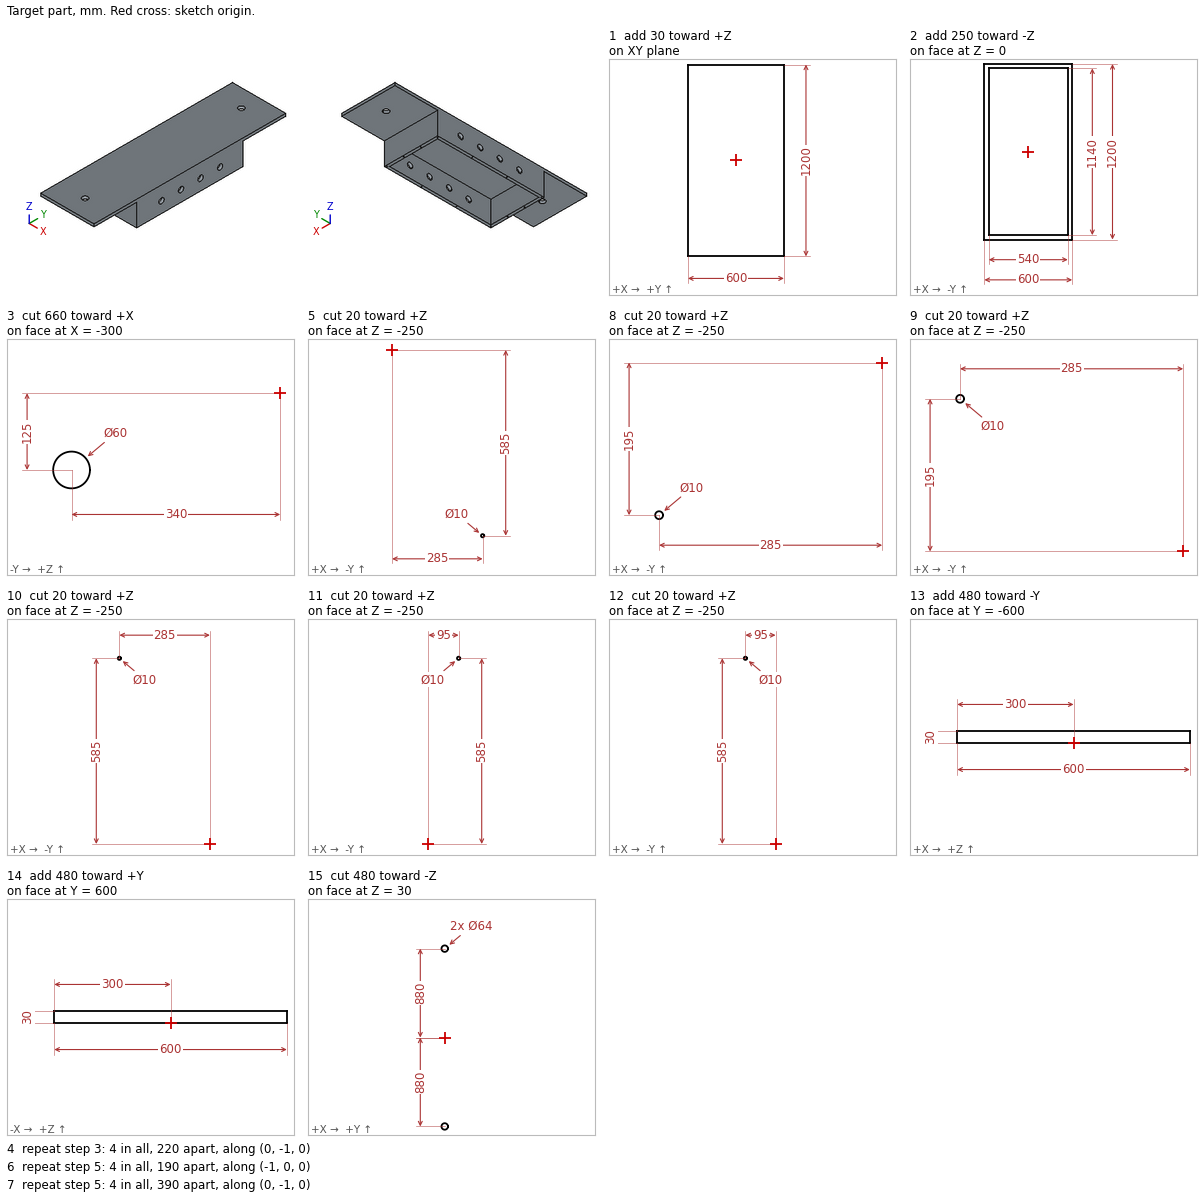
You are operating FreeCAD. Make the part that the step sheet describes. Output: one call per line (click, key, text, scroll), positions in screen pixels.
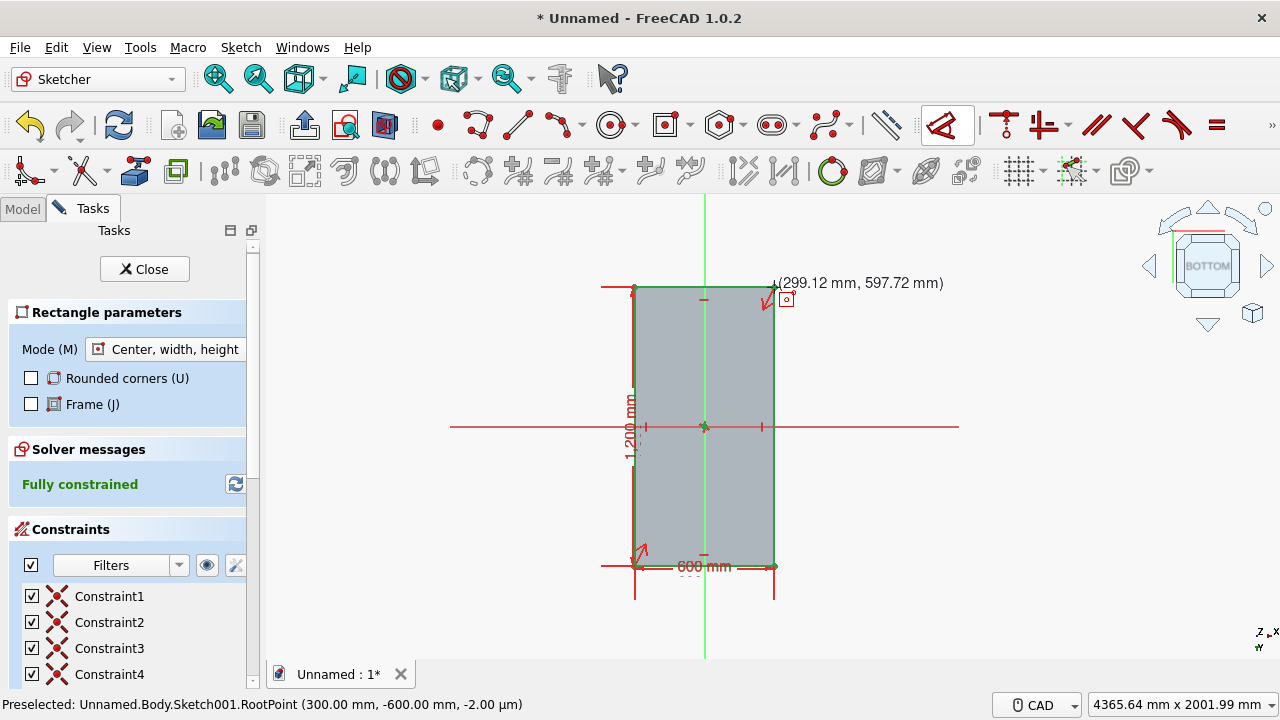
click(705, 427)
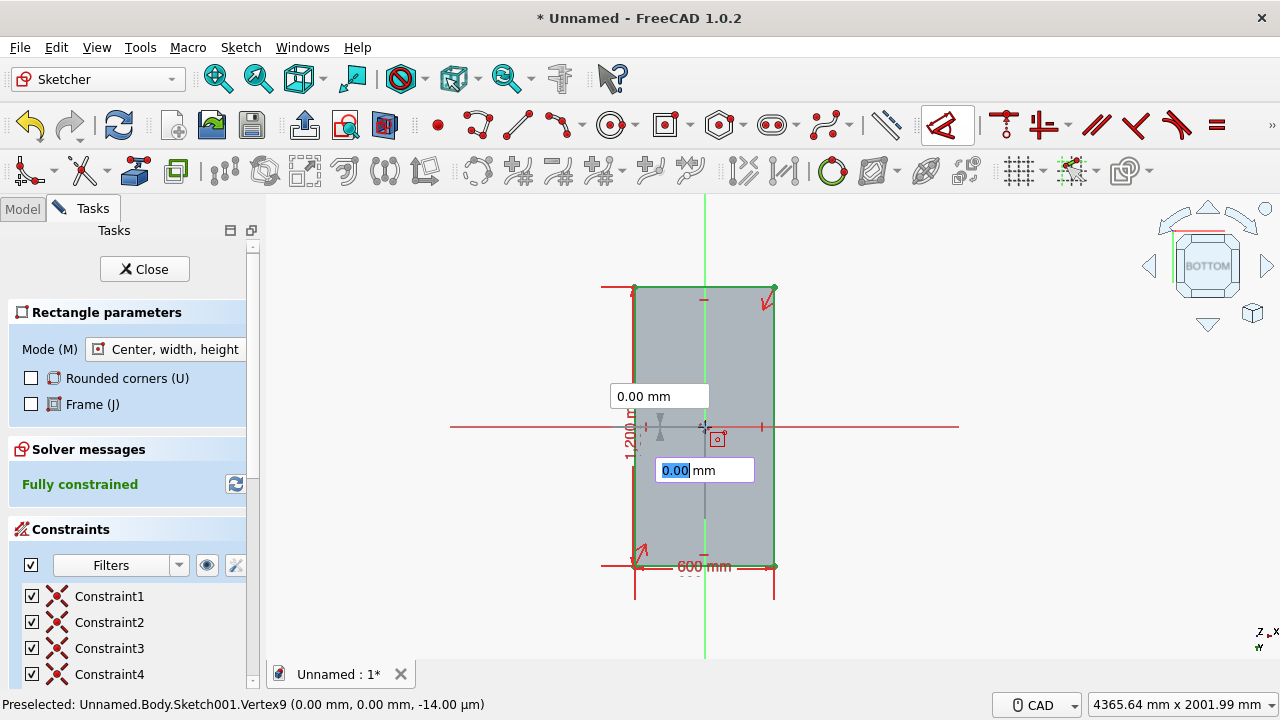
scroll(767, 294, up, 5)
move(767, 295)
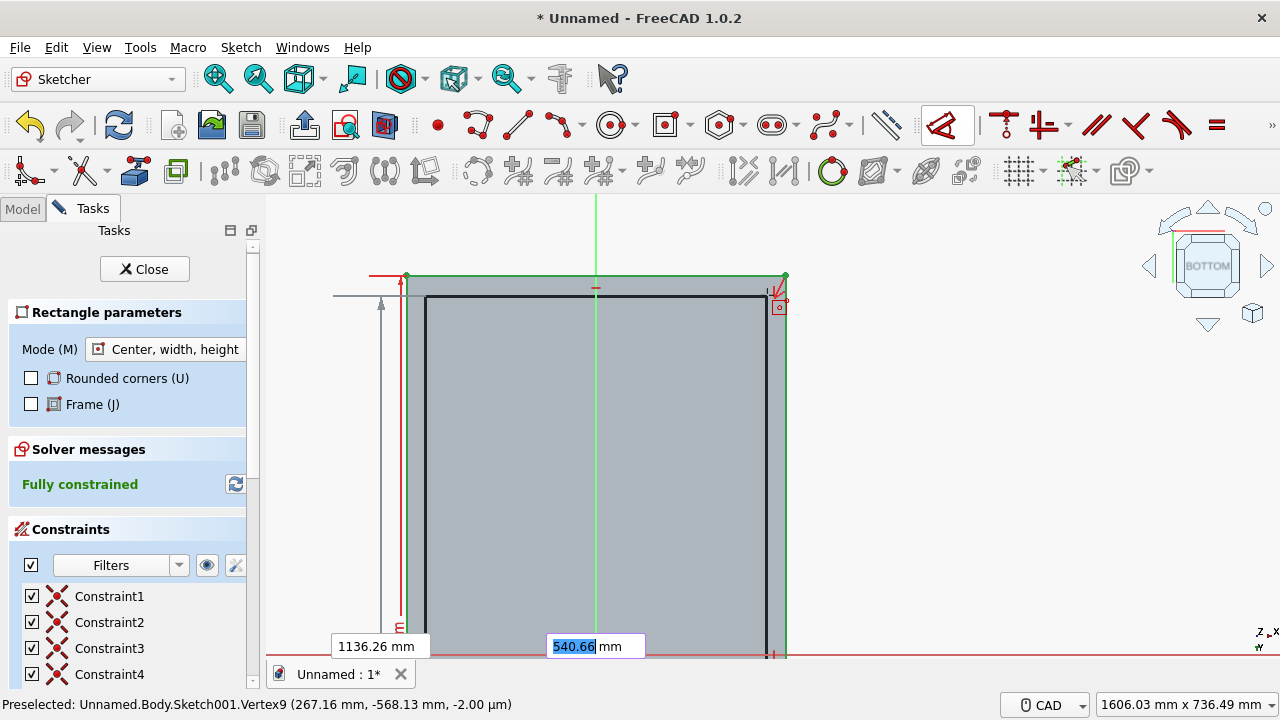
text(540)
key(Tab)
text(1140)
key(Return)
key(Escape)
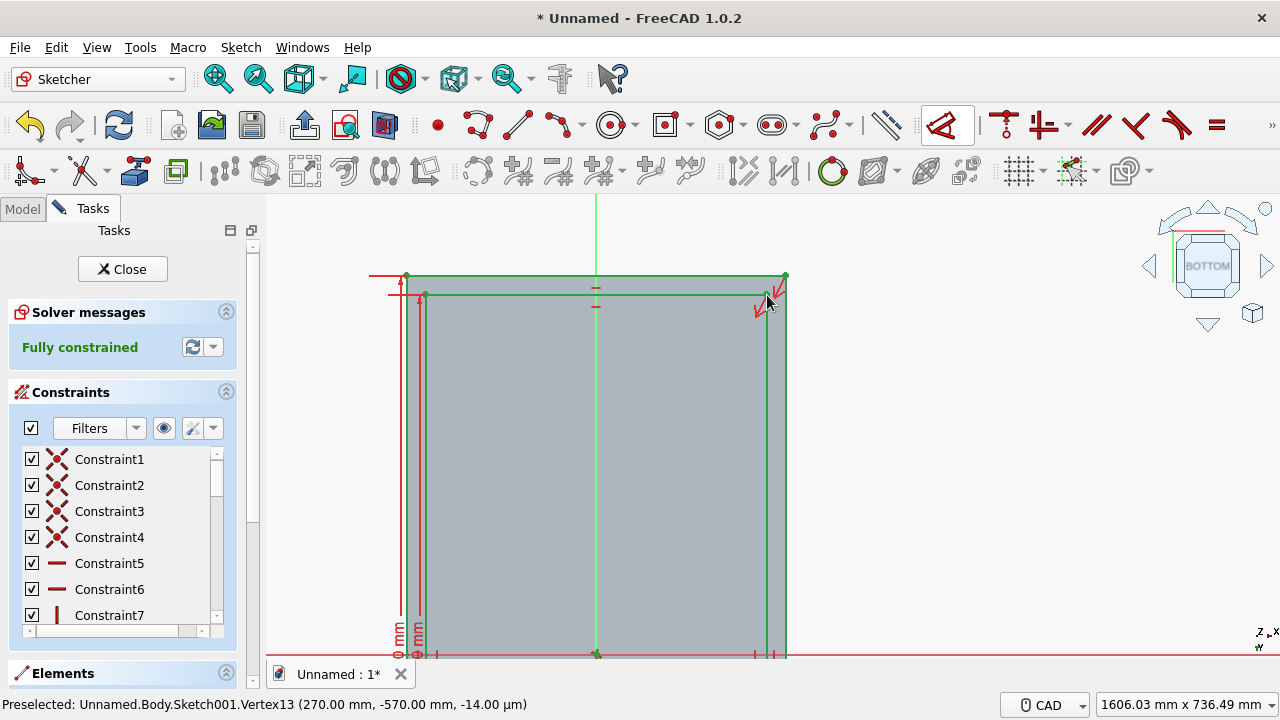
click(123, 269)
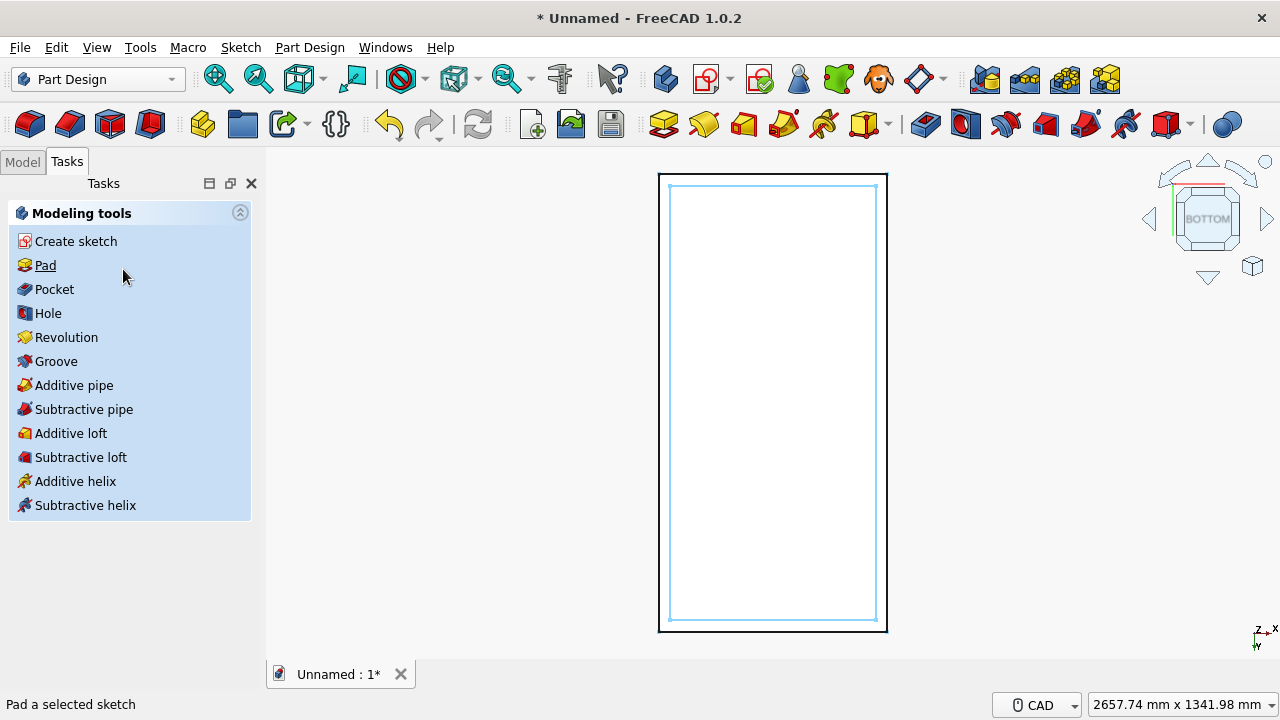
click(664, 124)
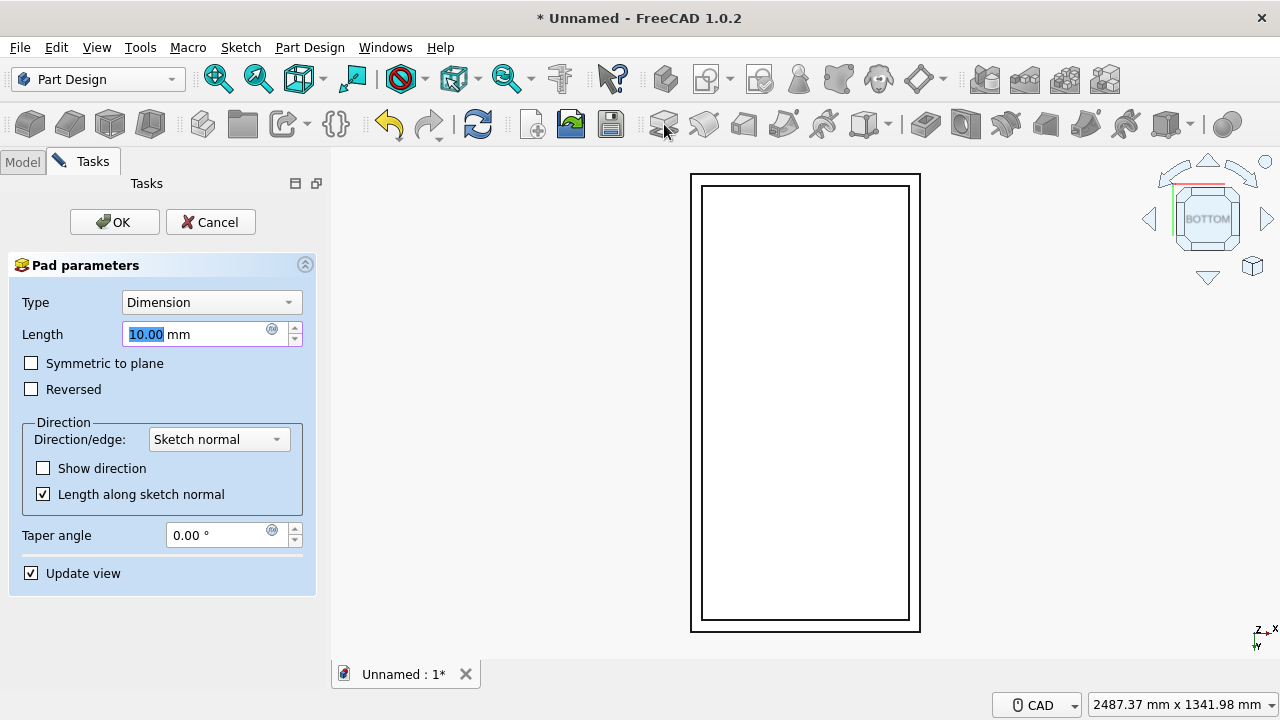
text(250)
key(Tab)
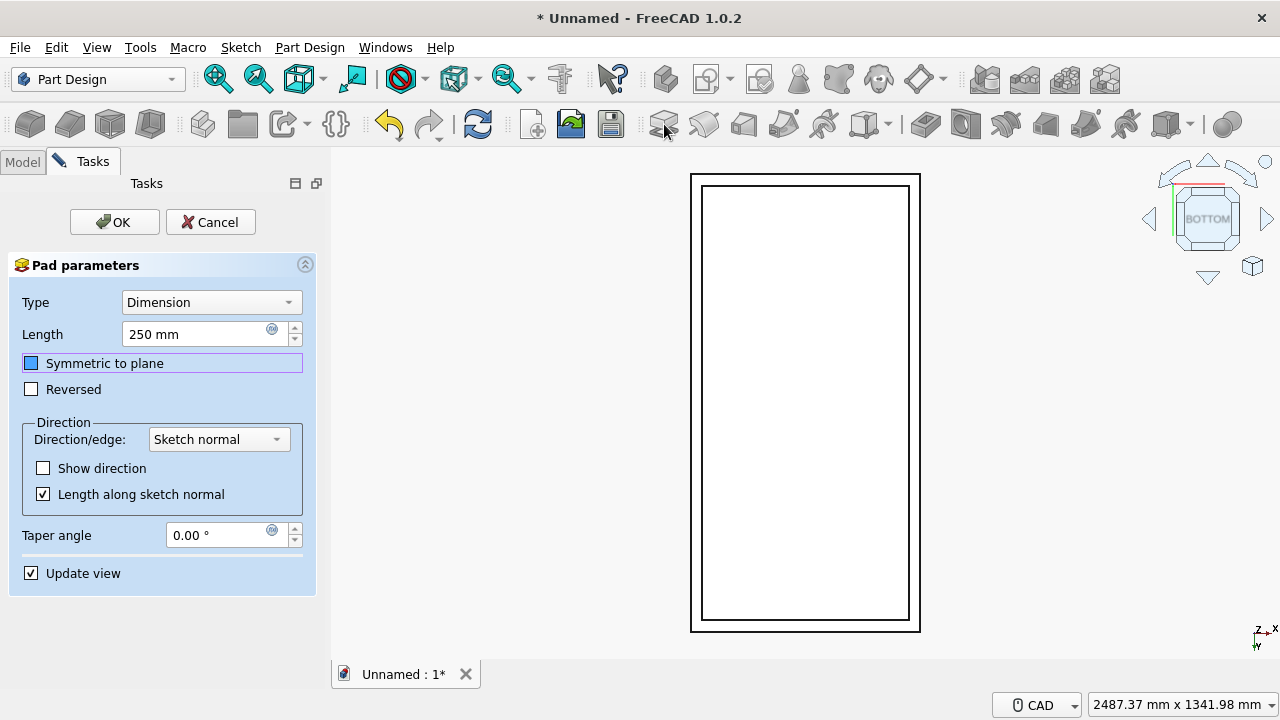
click(115, 222)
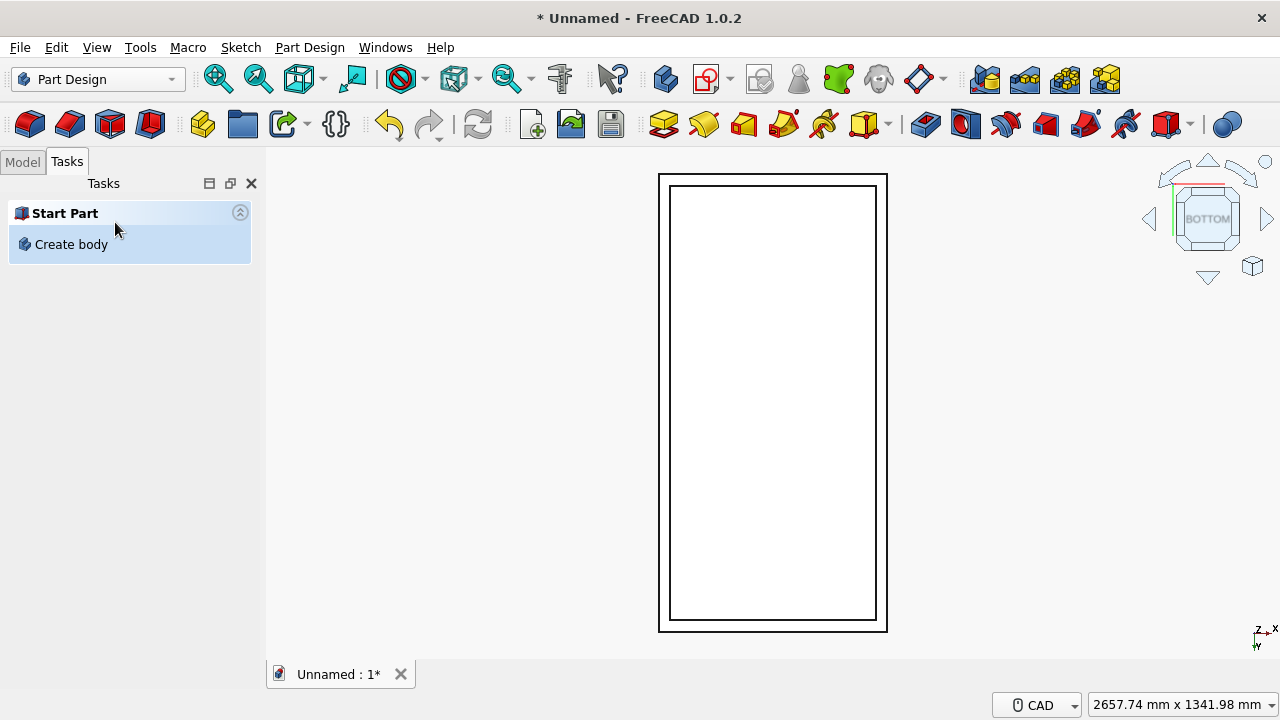
key(6)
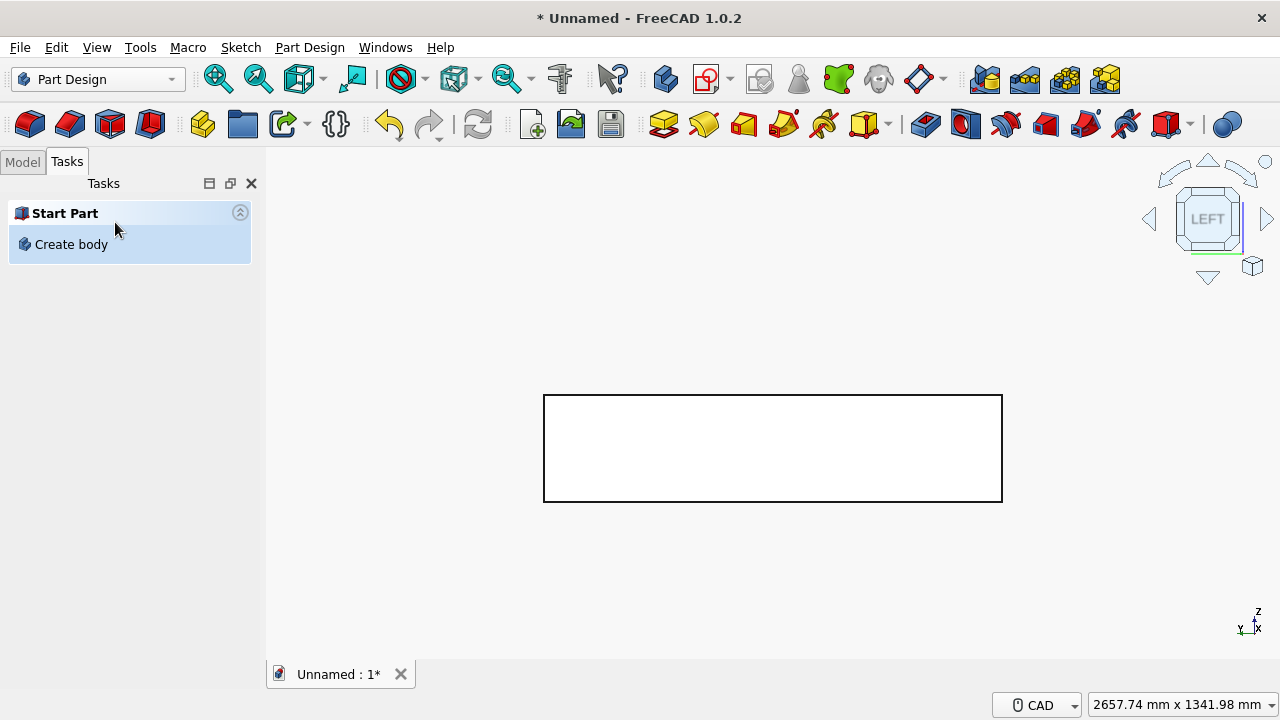
click(642, 448)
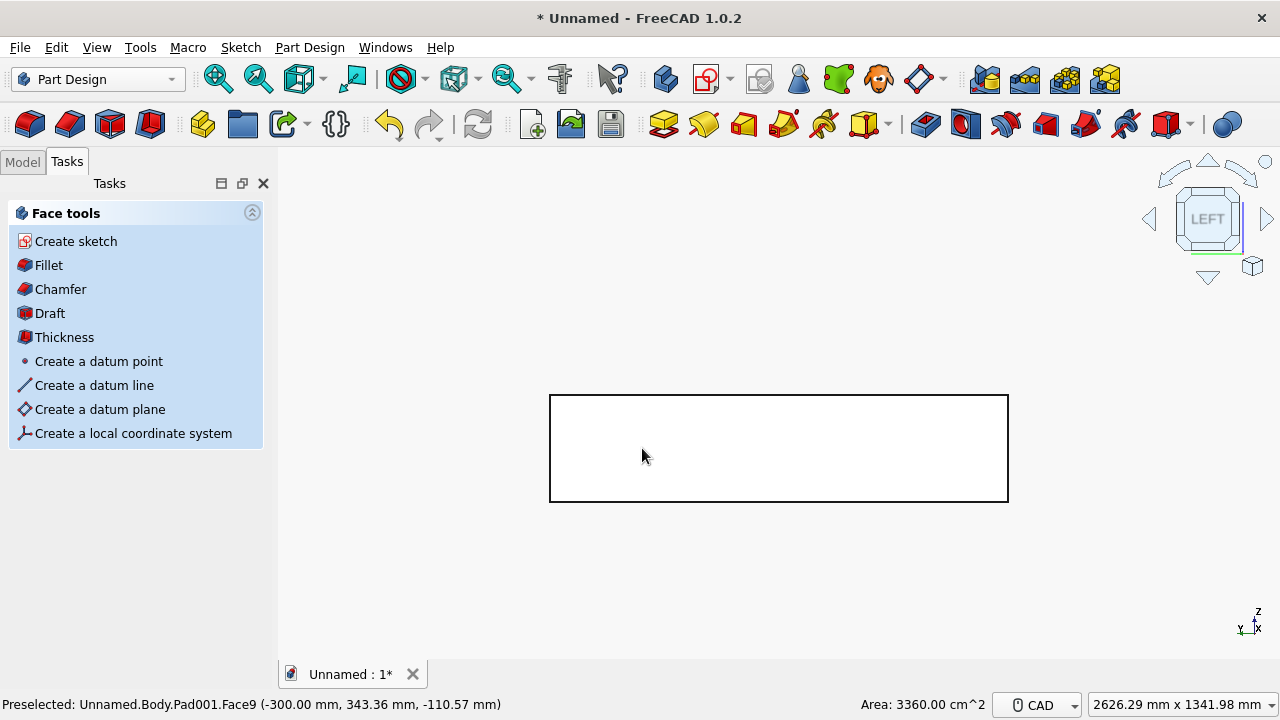
click(706, 80)